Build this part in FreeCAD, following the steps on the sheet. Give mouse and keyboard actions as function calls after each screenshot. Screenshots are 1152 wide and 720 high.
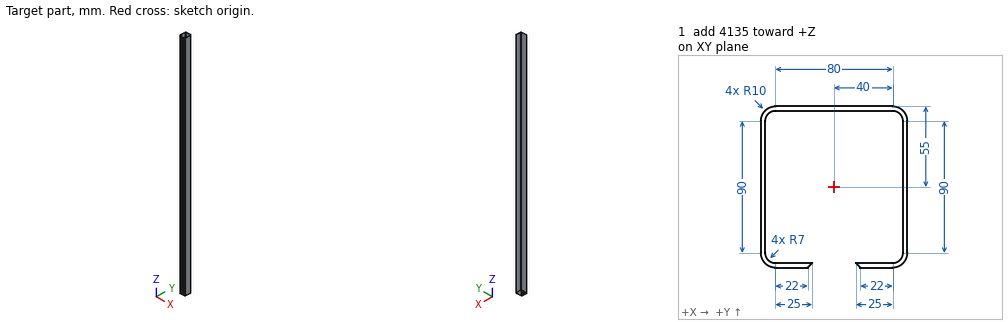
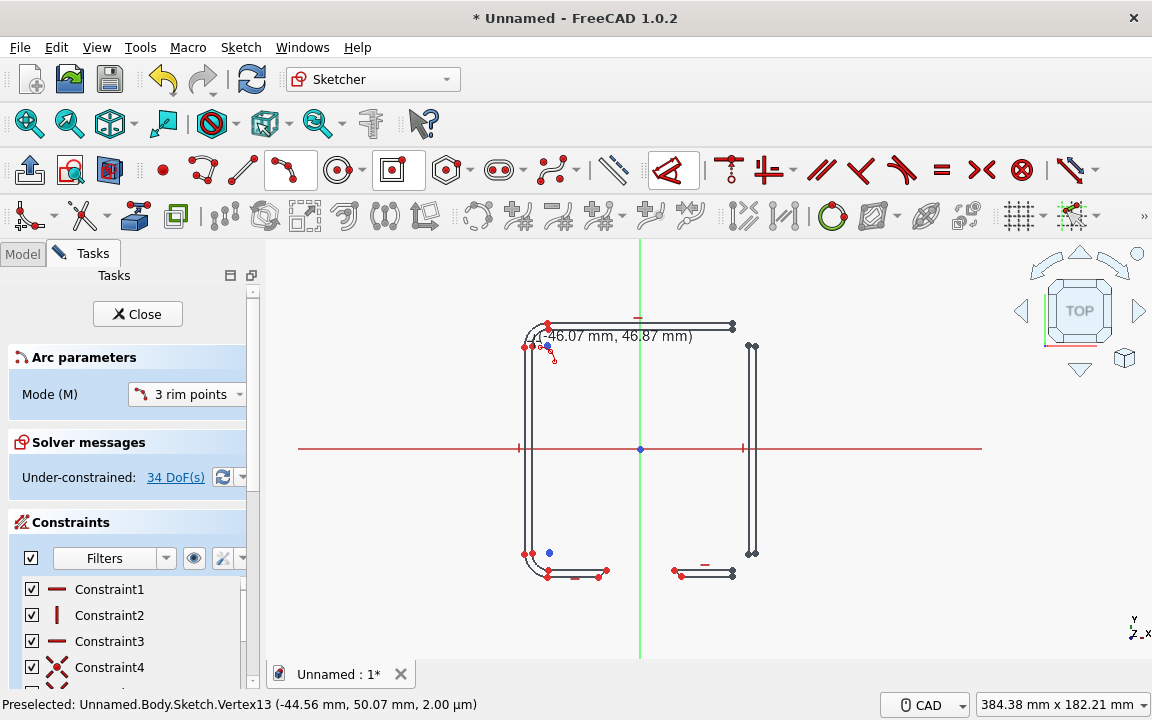
scroll(733, 330, up, 5)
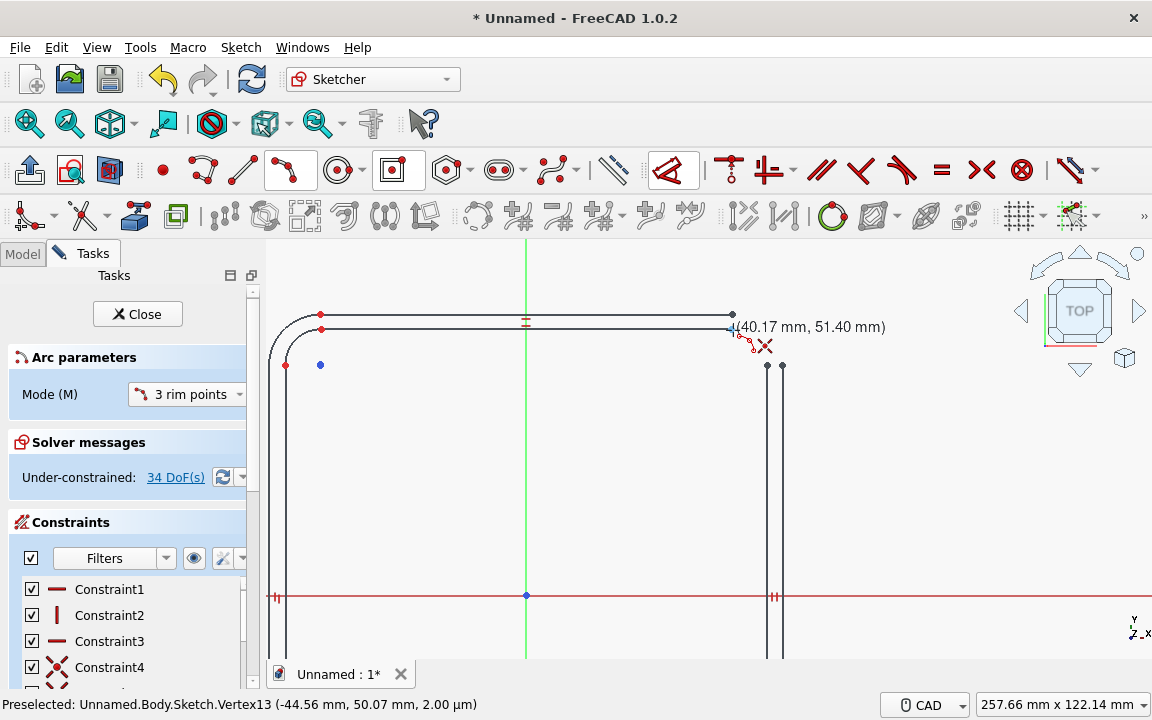
click(731, 329)
click(774, 373)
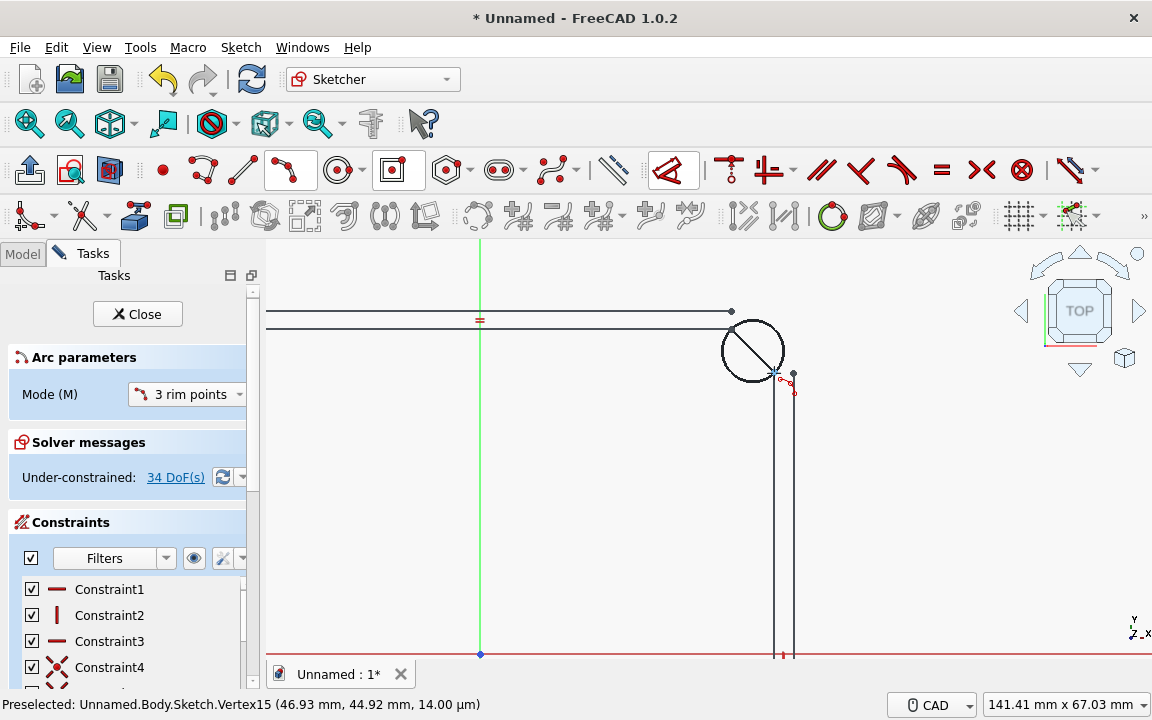
scroll(762, 341, up, 2)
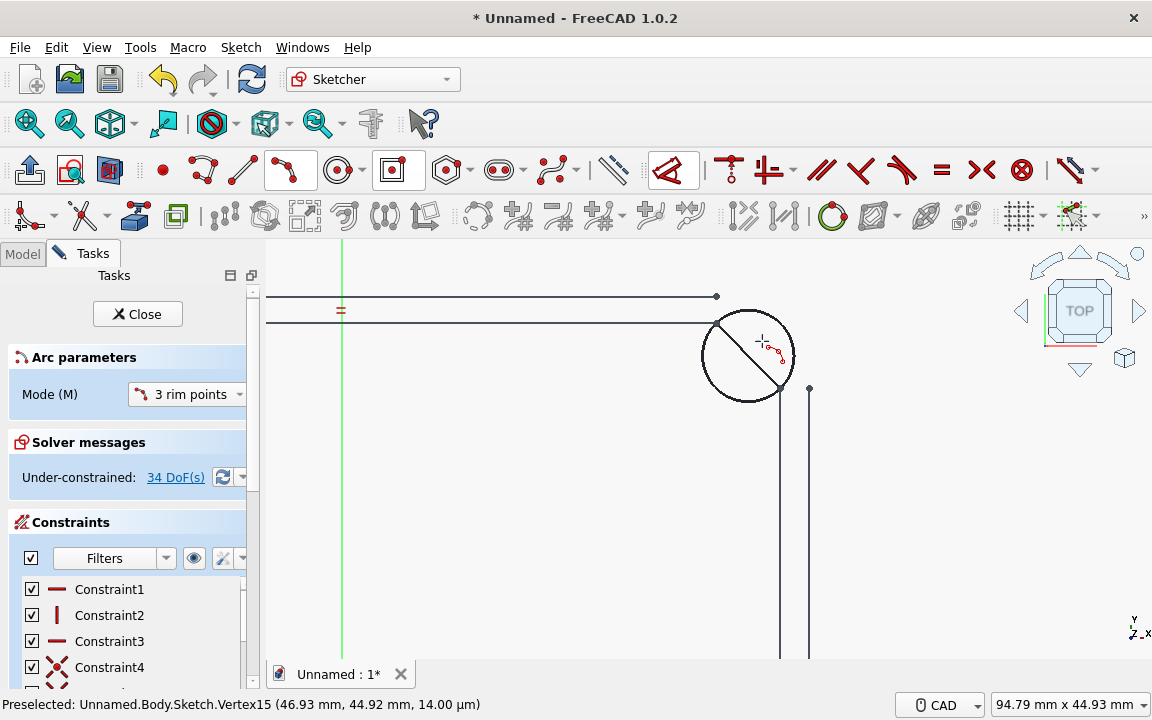
click(762, 341)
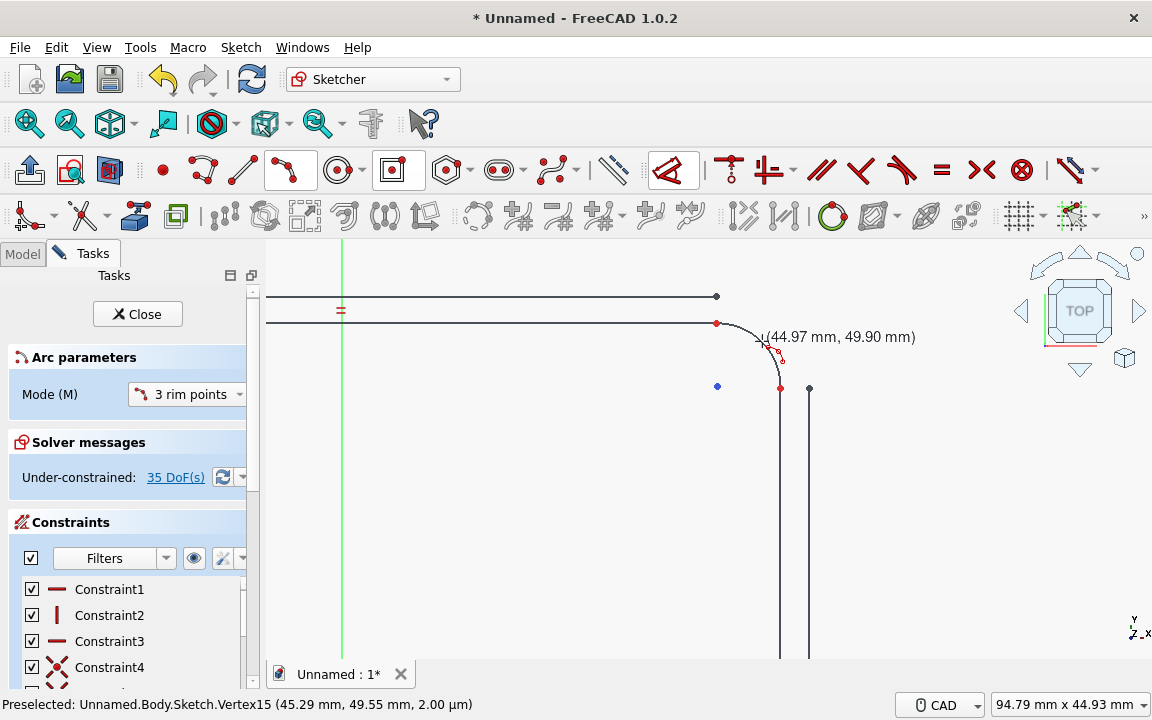
scroll(738, 331, down, 7)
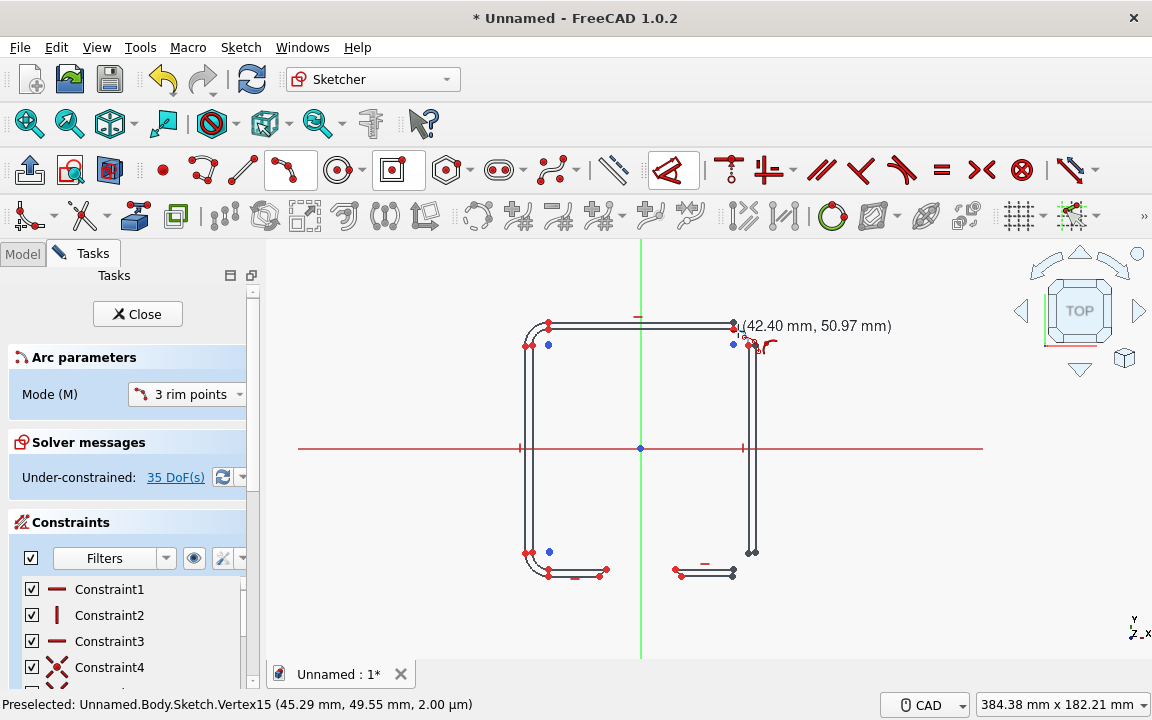
scroll(749, 553, up, 5)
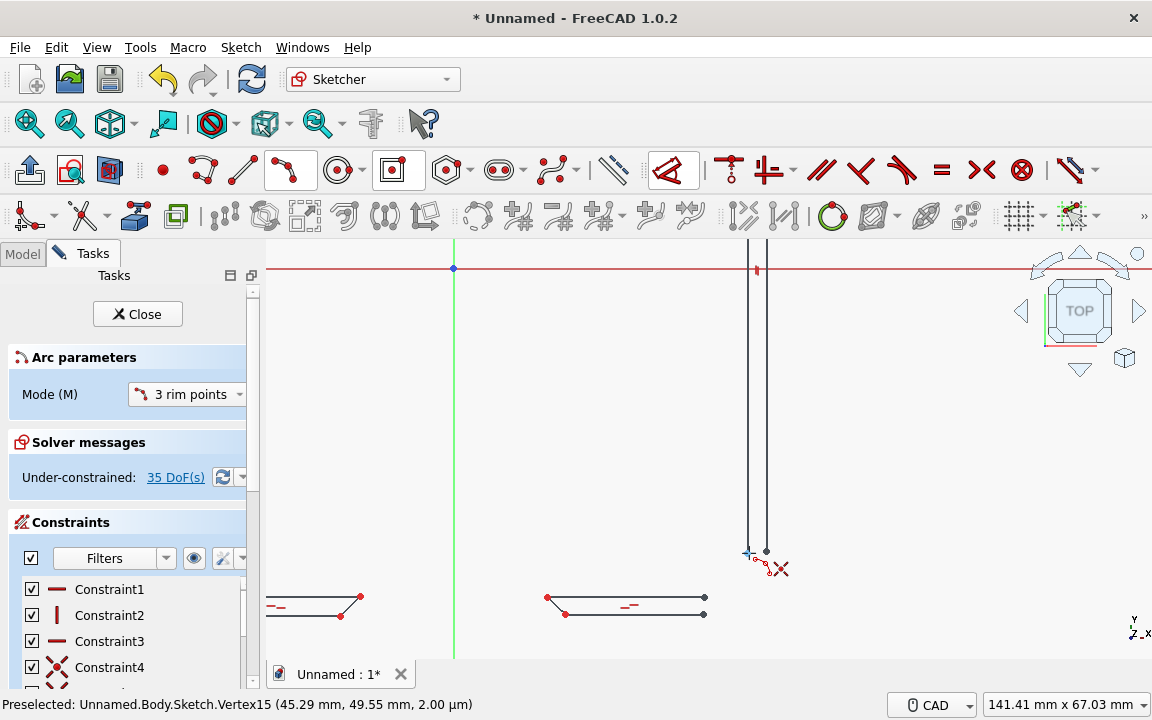
click(748, 554)
click(705, 597)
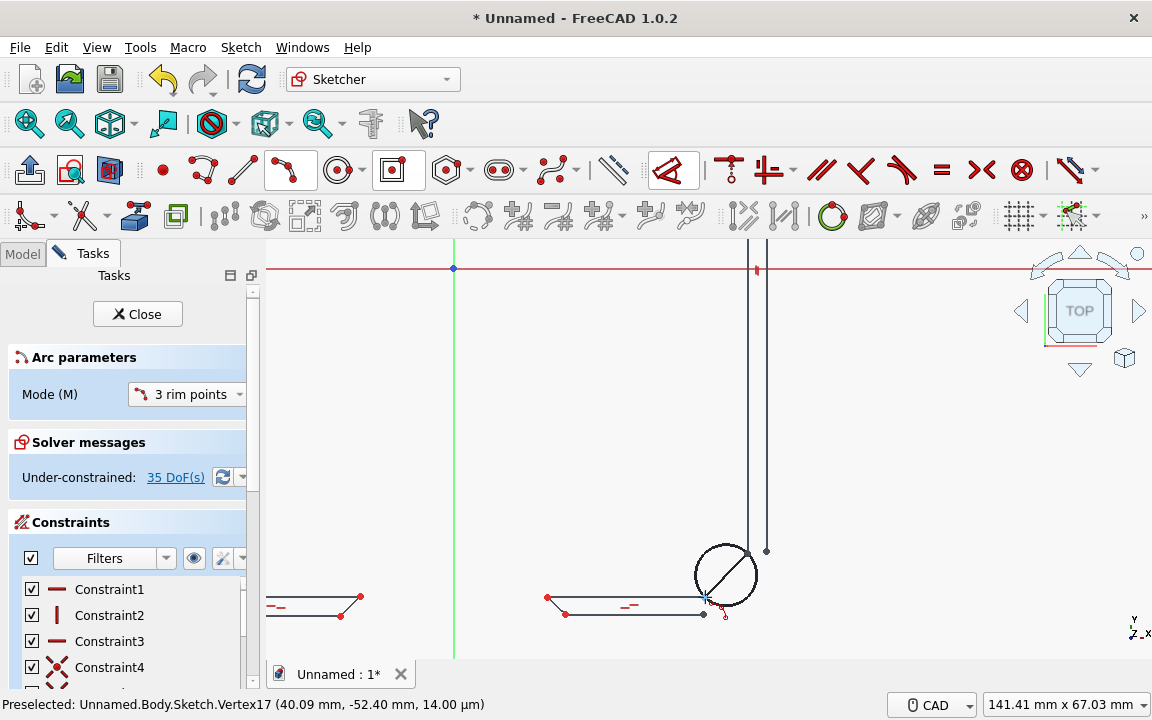
scroll(735, 582, up, 2)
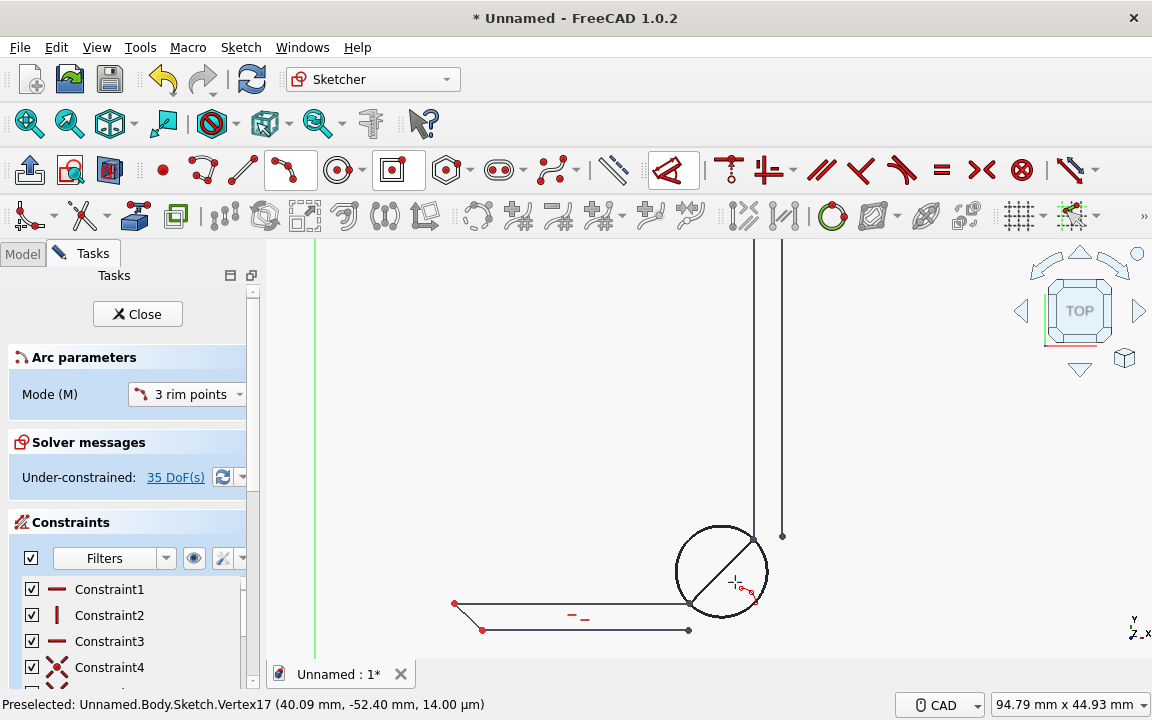
click(735, 581)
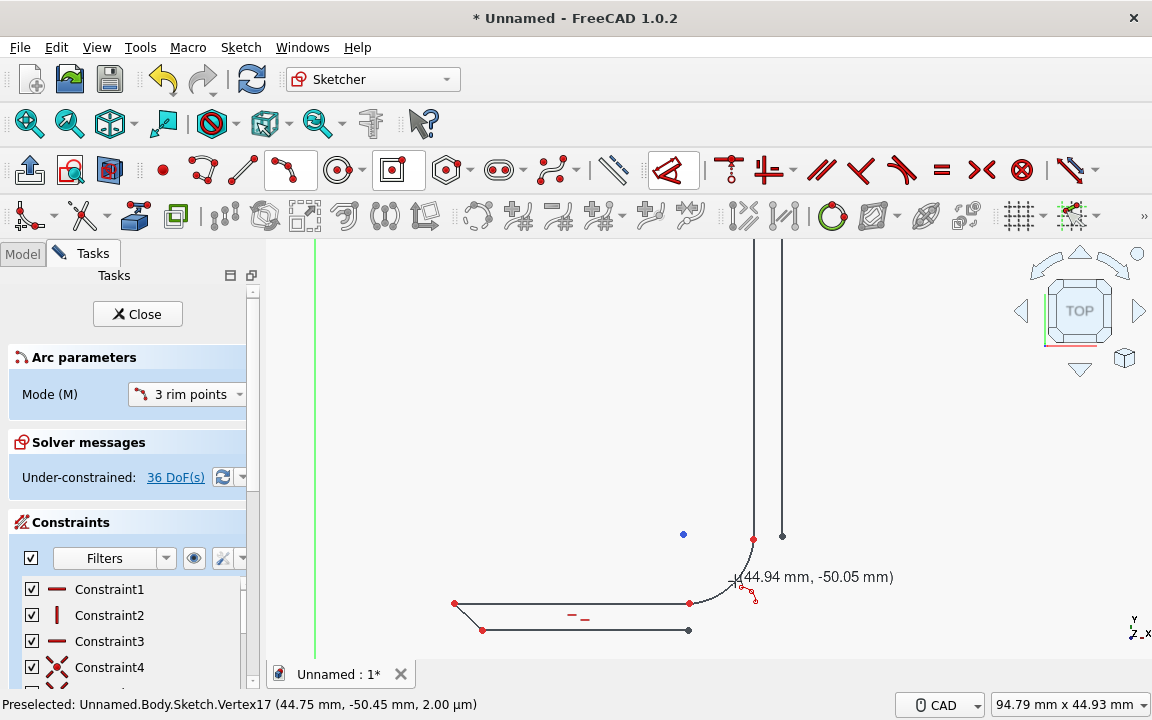
click(688, 630)
click(782, 536)
click(755, 601)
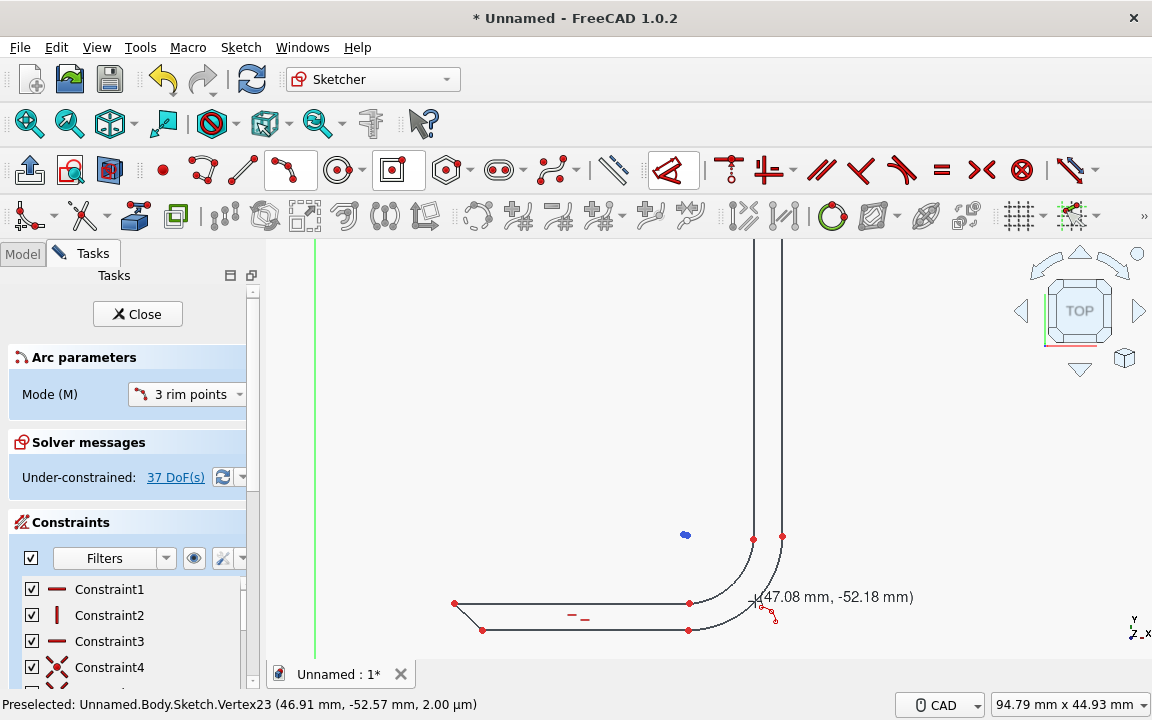
scroll(747, 559, down, 7)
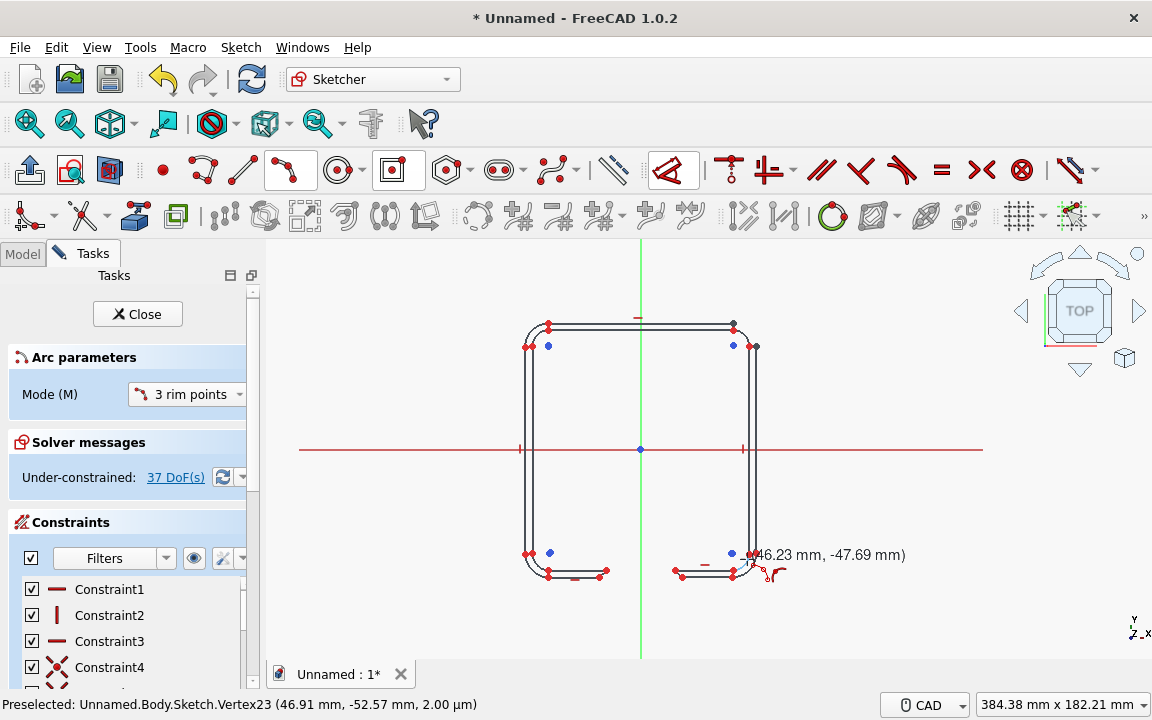
scroll(756, 346, up, 5)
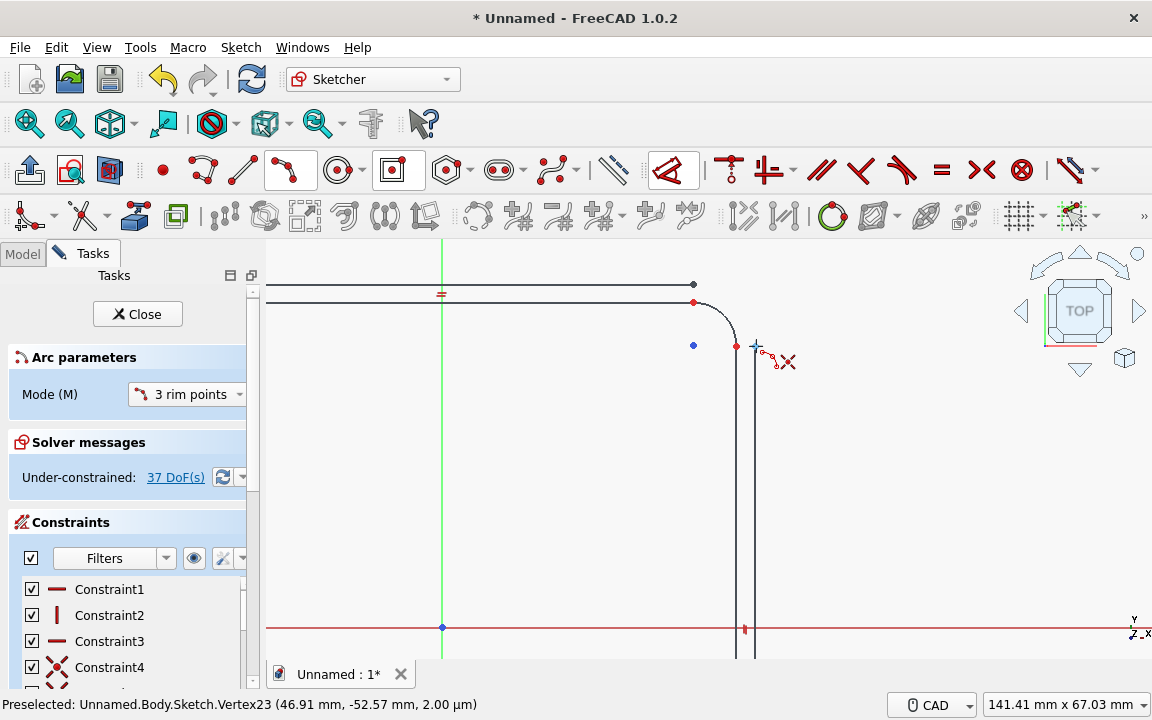
click(755, 347)
click(693, 285)
click(737, 302)
key(Escape)